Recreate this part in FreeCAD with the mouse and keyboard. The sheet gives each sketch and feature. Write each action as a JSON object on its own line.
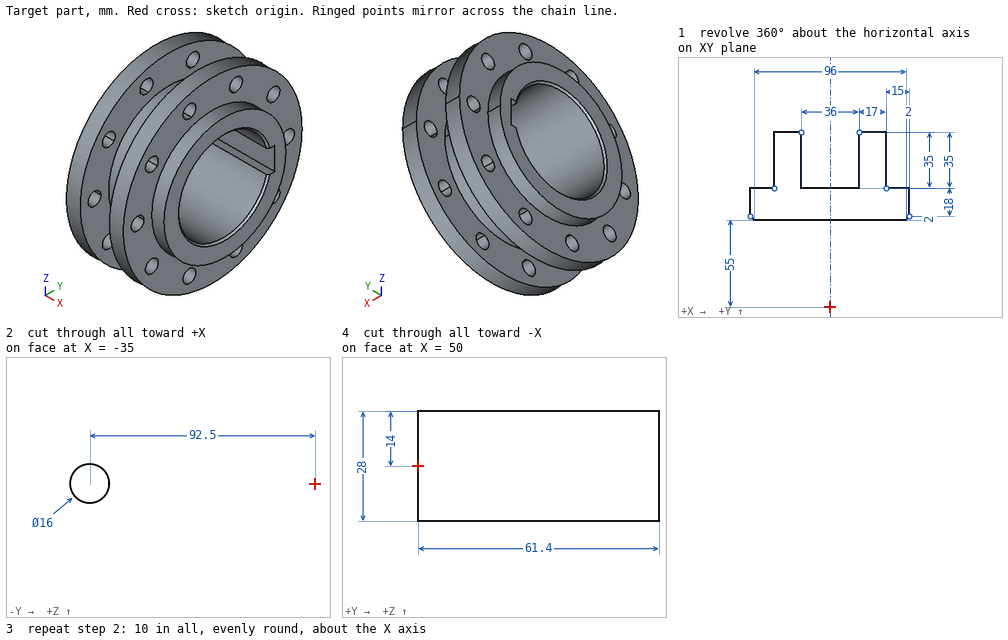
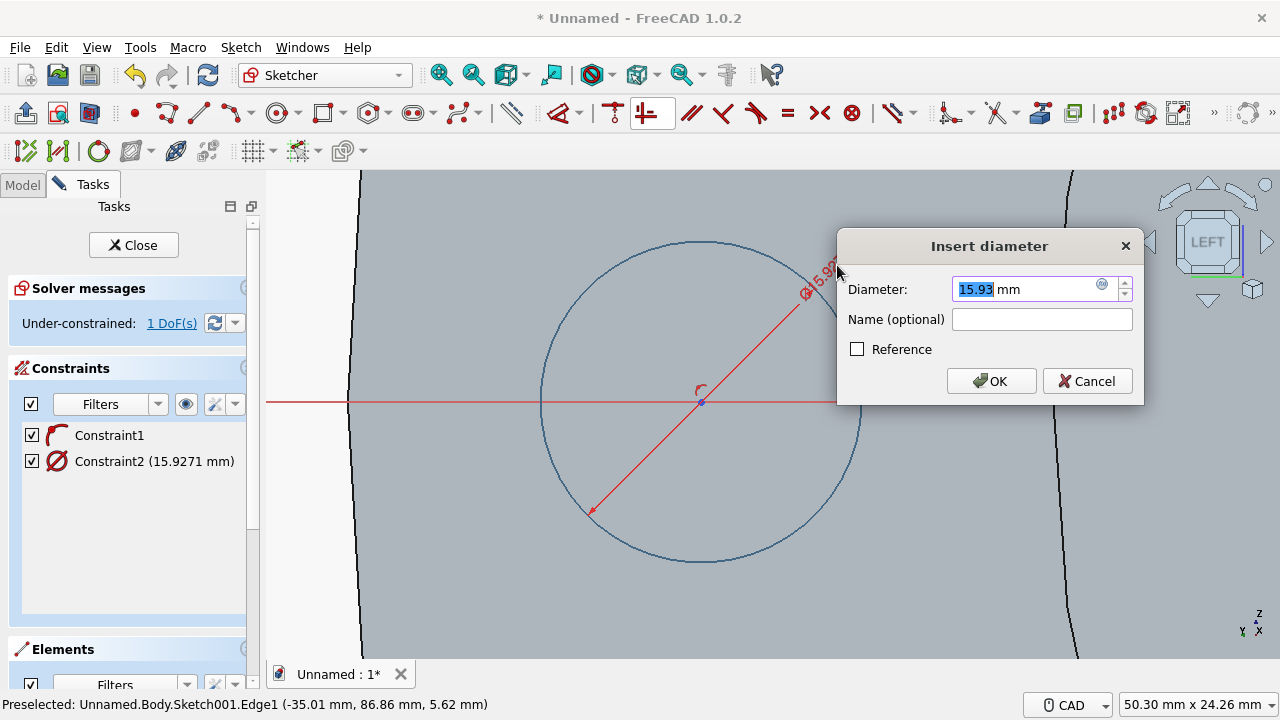
{"action": "type", "text": "16"}
{"action": "key", "text": "Return"}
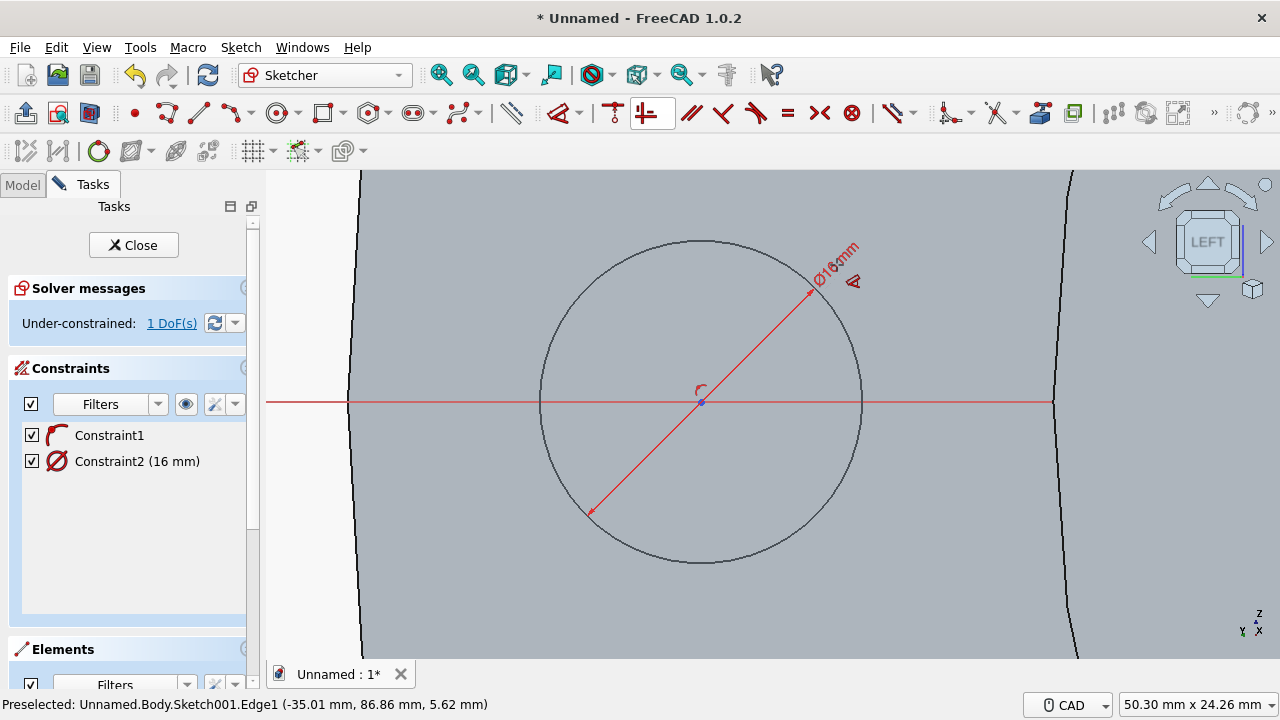
{"action": "left_click", "coordinate": [701, 402]}
{"action": "left_click", "coordinate": [908, 436]}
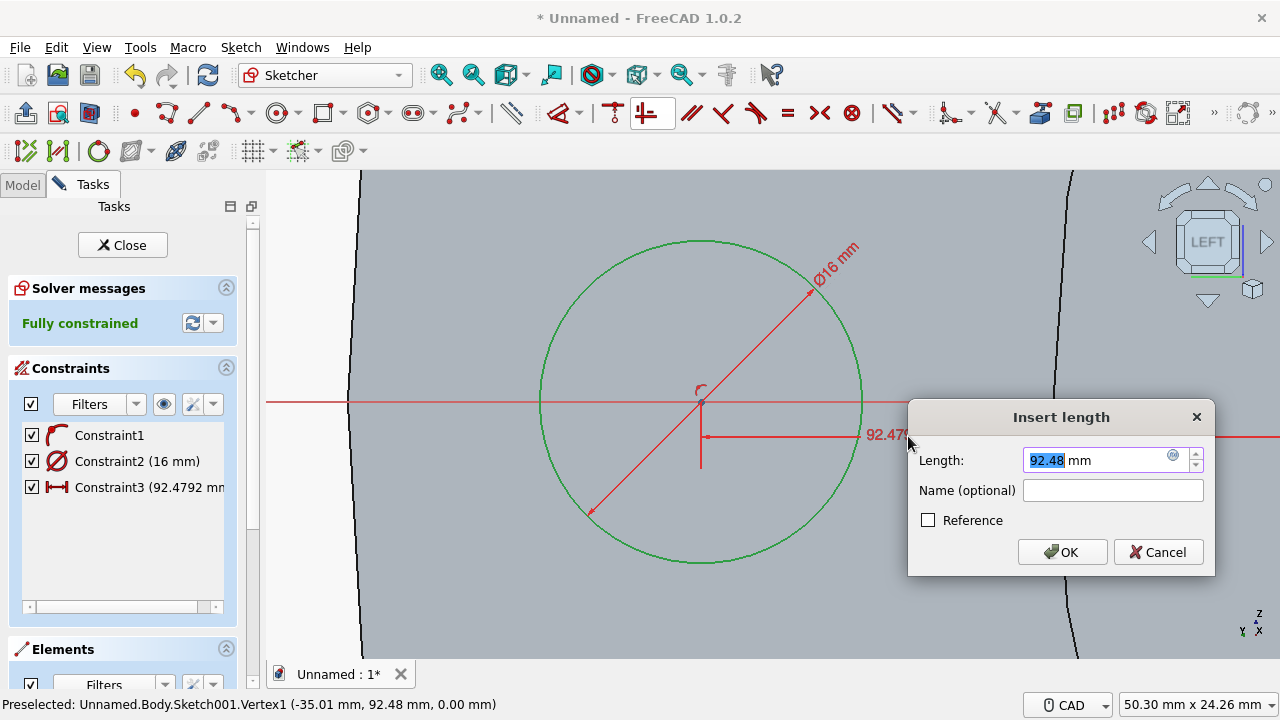
{"action": "type", "text": "92.5"}
{"action": "key", "text": "Return"}
{"action": "key", "text": "Escape"}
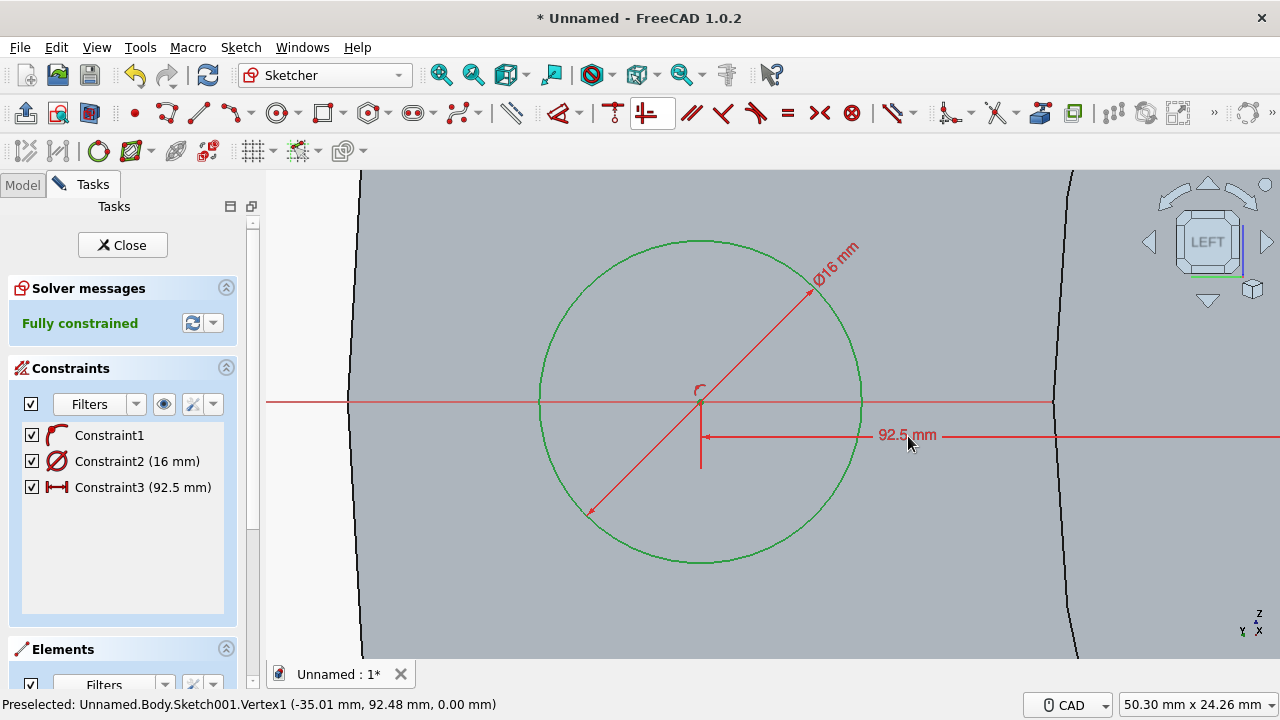
{"action": "left_click", "coordinate": [123, 245]}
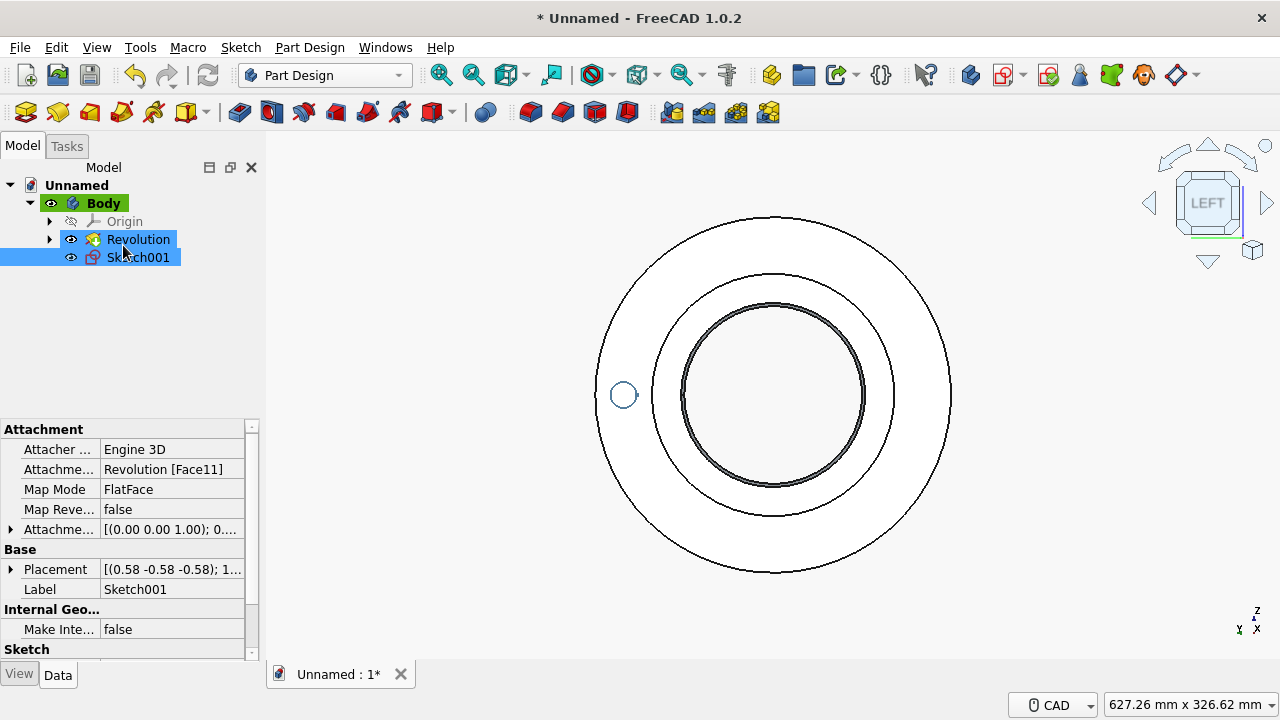
{"action": "left_click", "coordinate": [240, 112]}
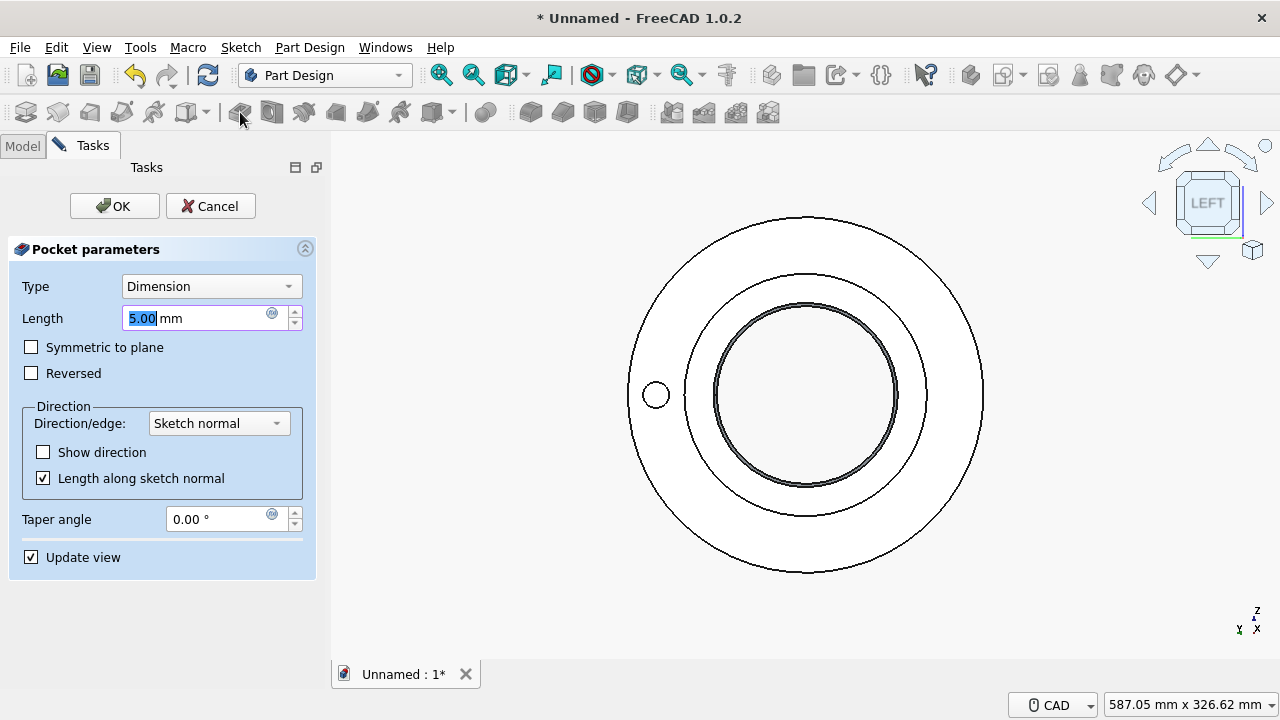
{"action": "left_click", "coordinate": [212, 286]}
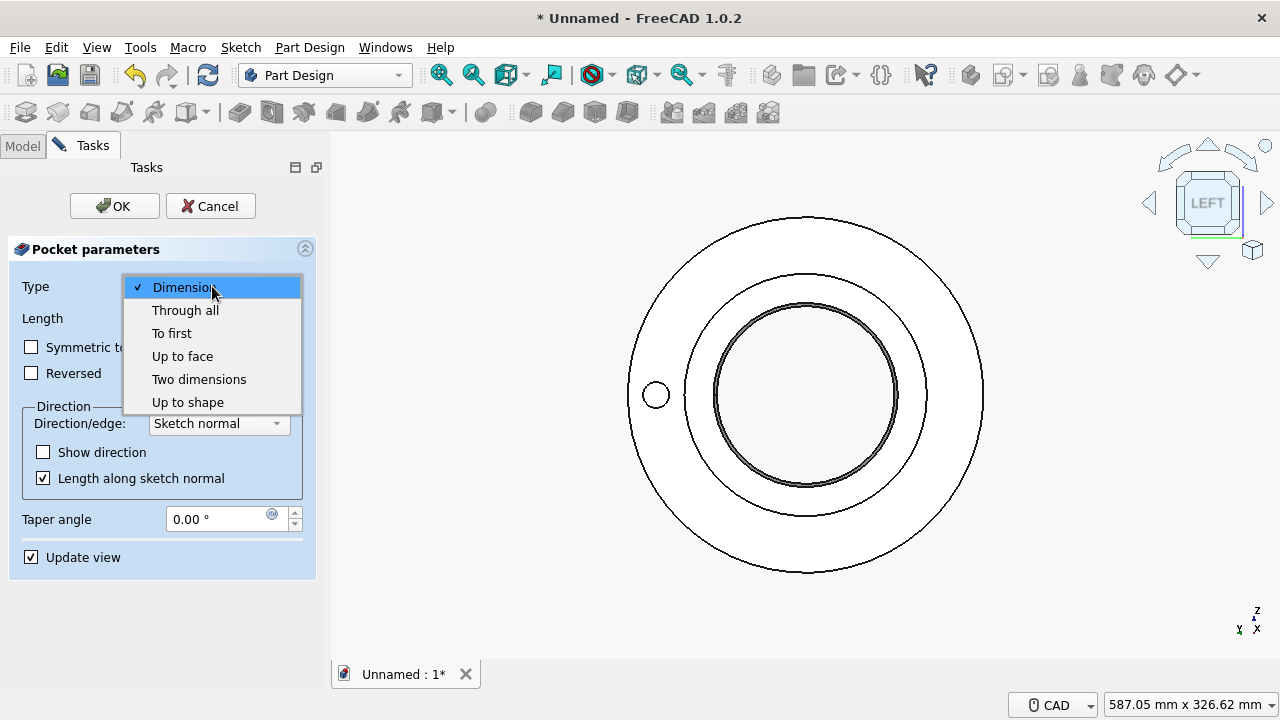
{"action": "left_click", "coordinate": [212, 310]}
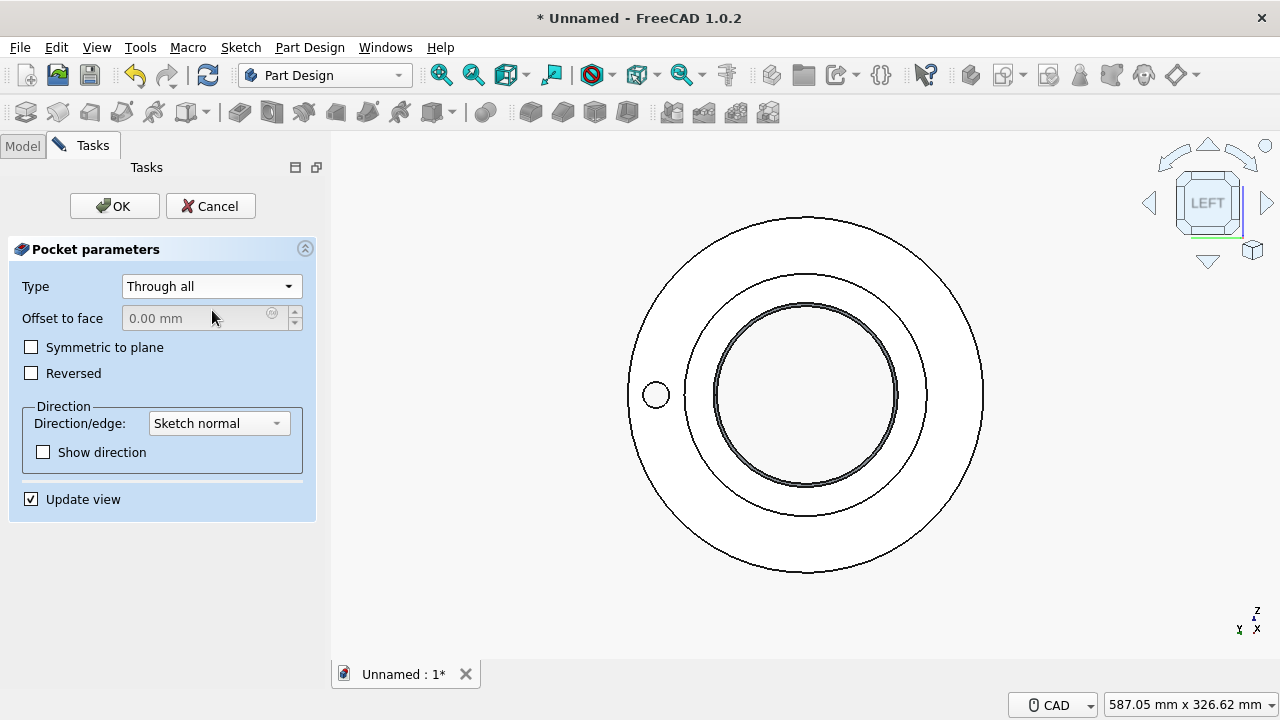
{"action": "left_click", "coordinate": [115, 206]}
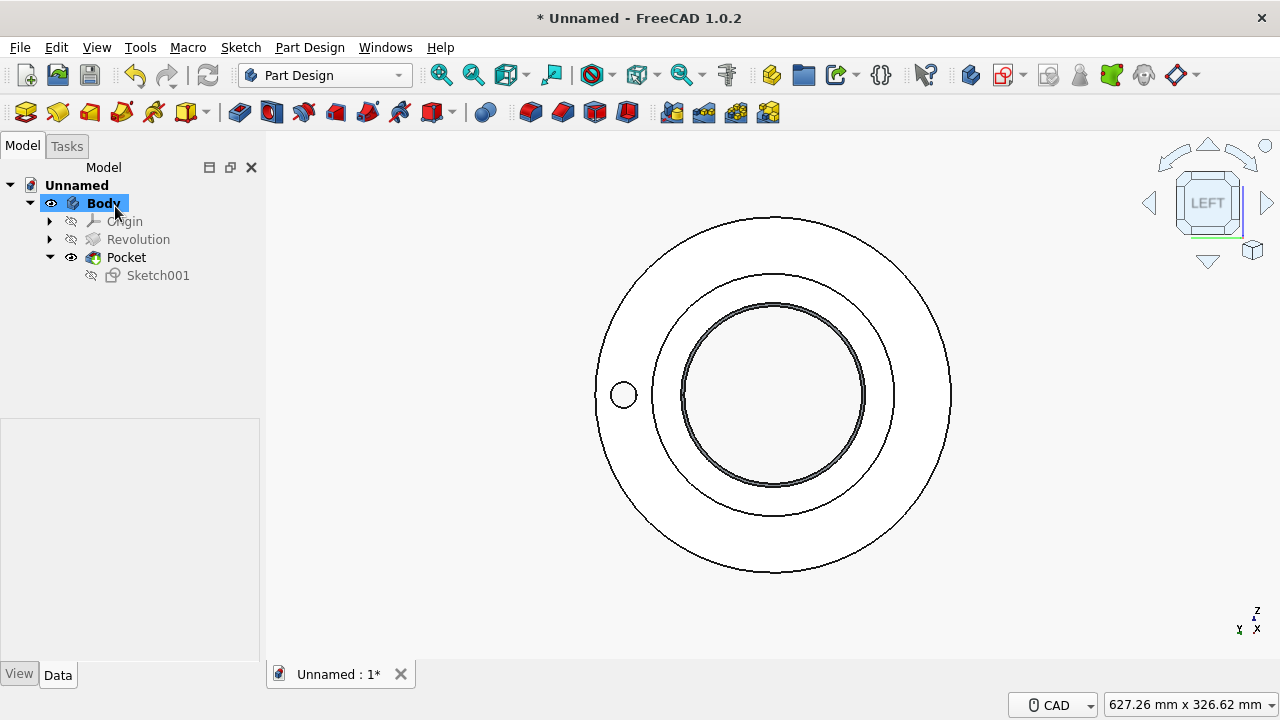
{"action": "left_click", "coordinate": [116, 257]}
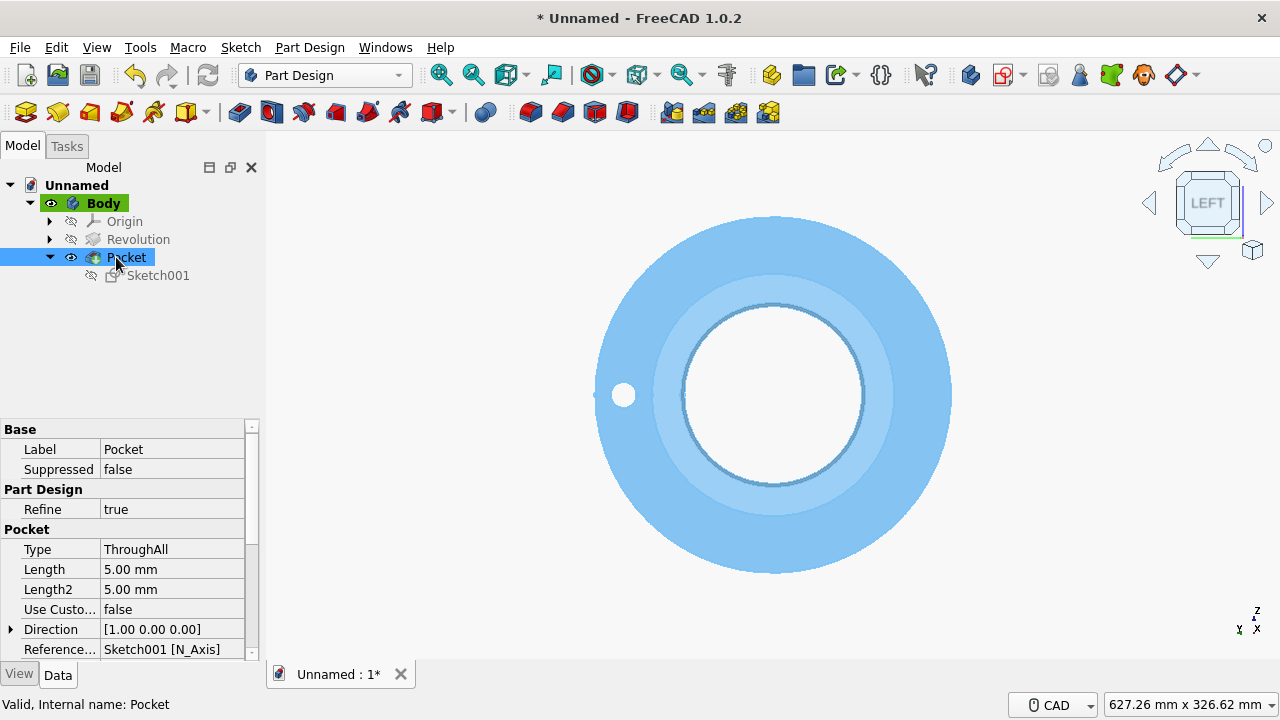
{"action": "left_click", "coordinate": [736, 112]}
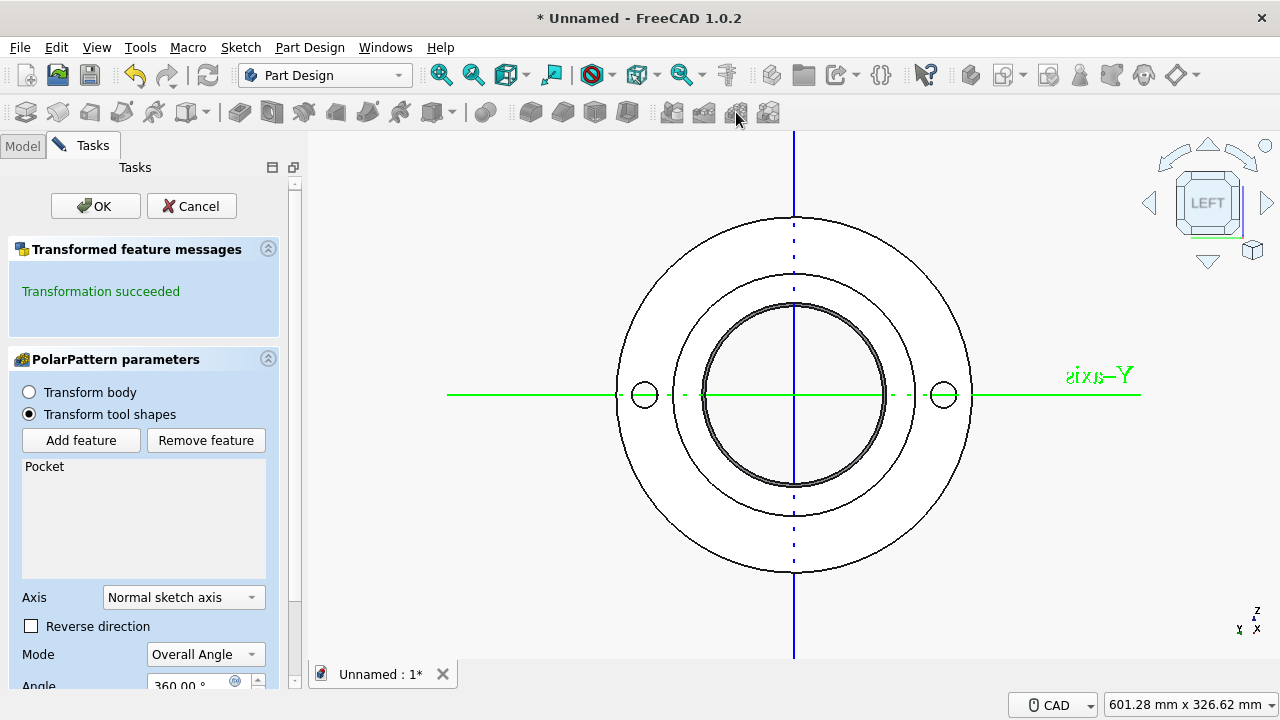
{"action": "left_click", "coordinate": [184, 598]}